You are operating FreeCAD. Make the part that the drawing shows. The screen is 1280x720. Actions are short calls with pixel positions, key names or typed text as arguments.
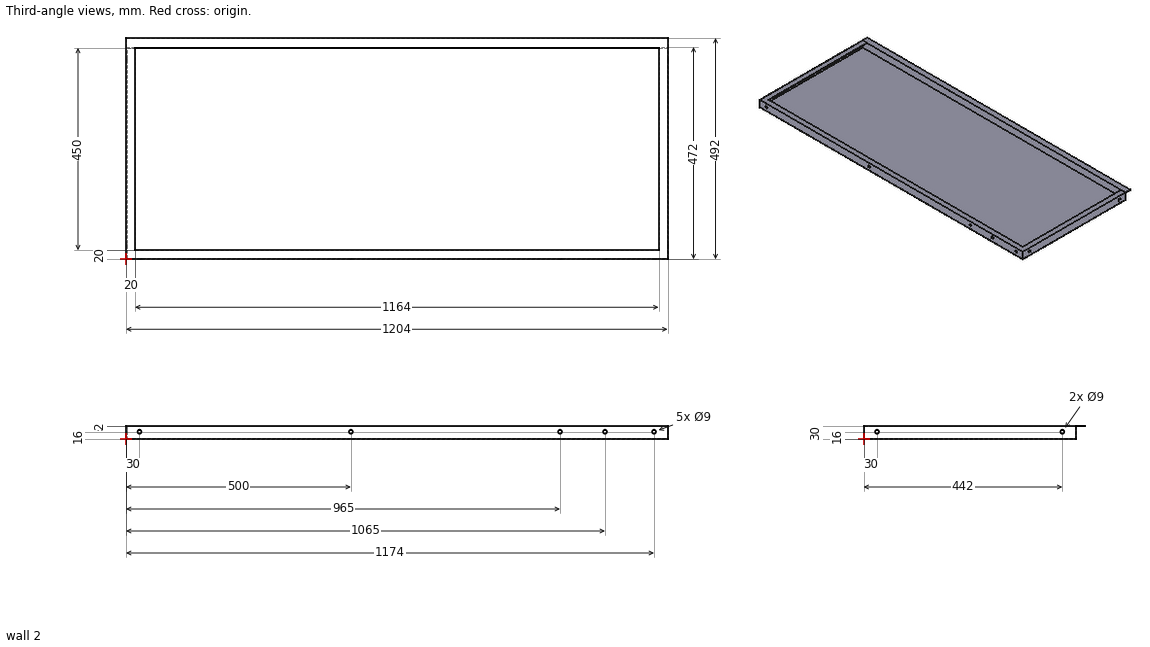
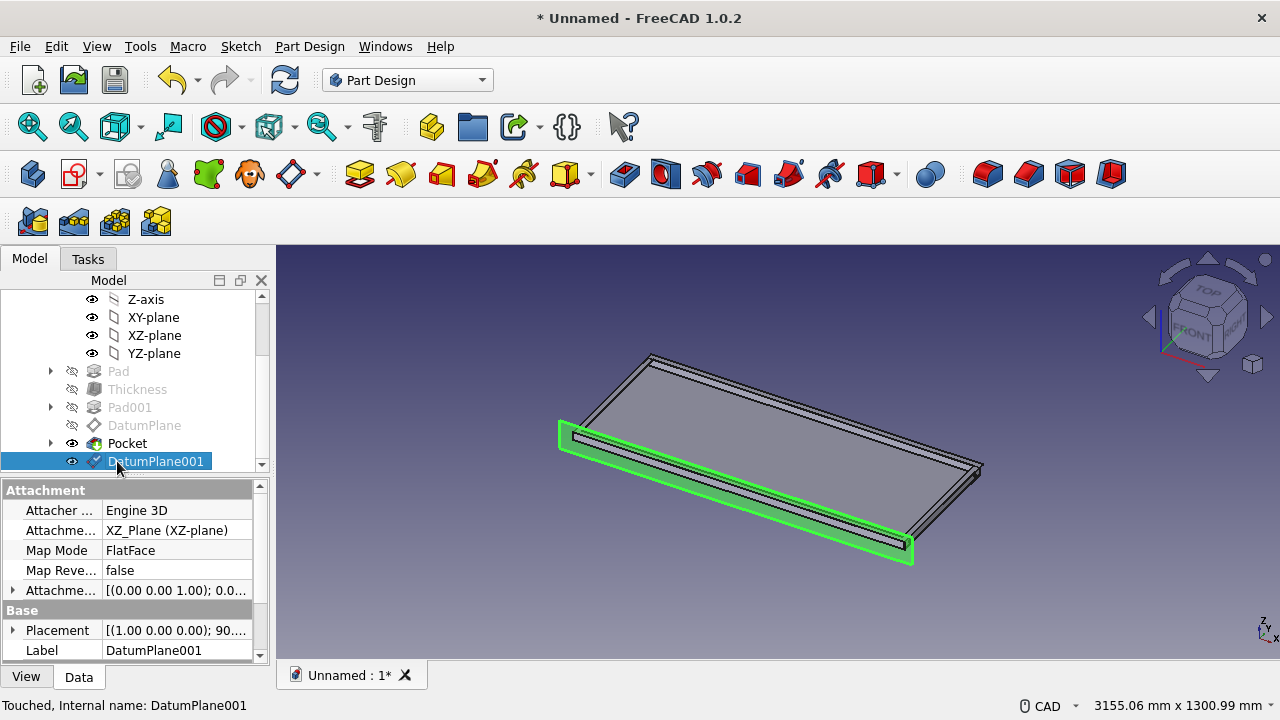
click(74, 174)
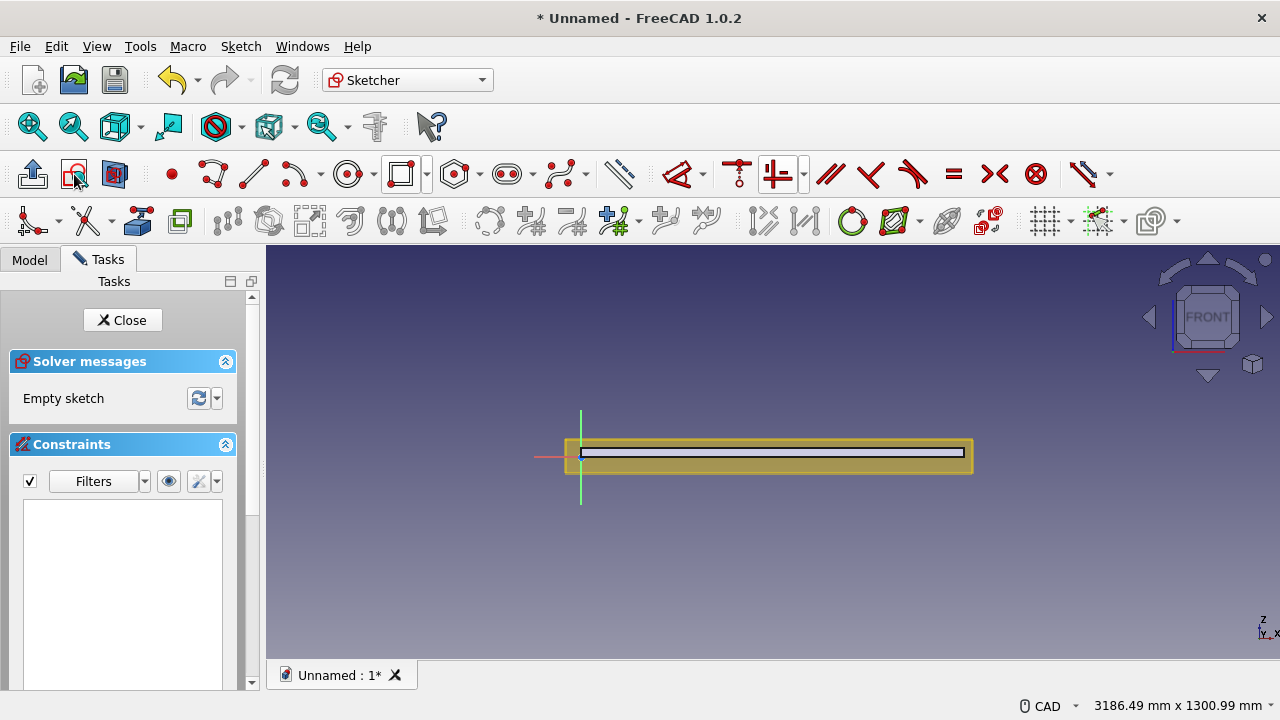
key(q)
key(s)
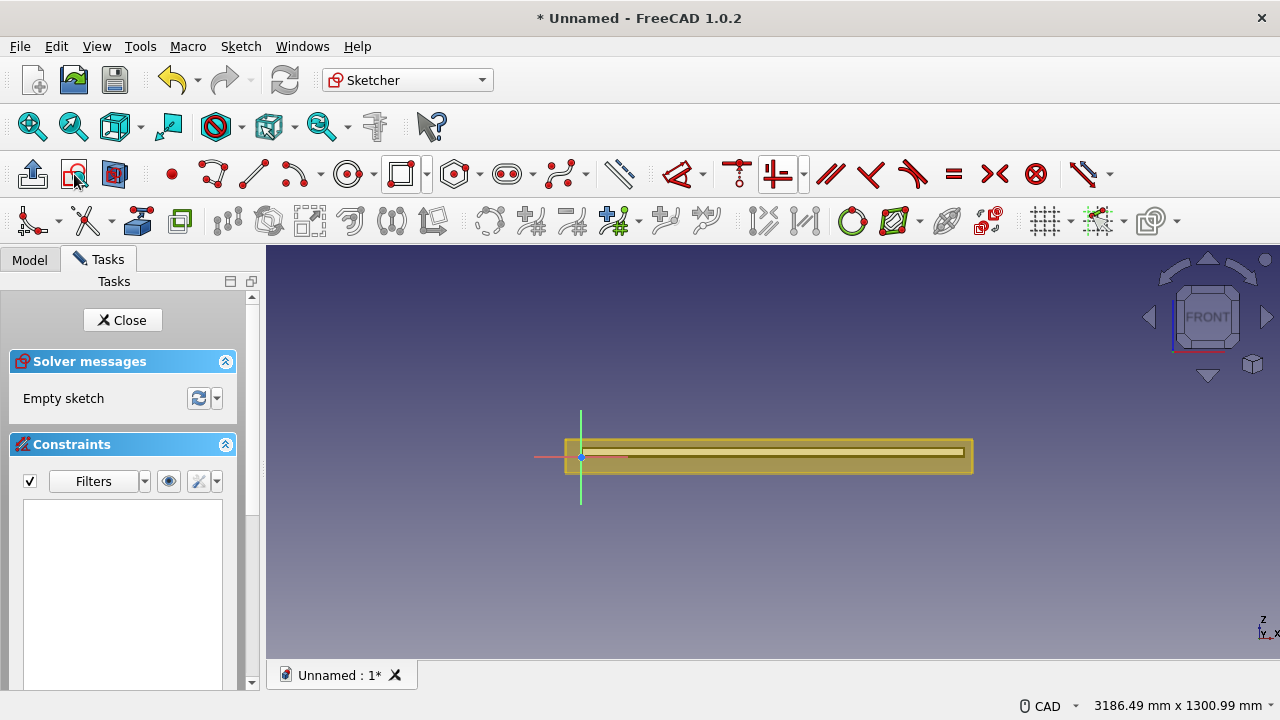
scroll(899, 458, up, 2)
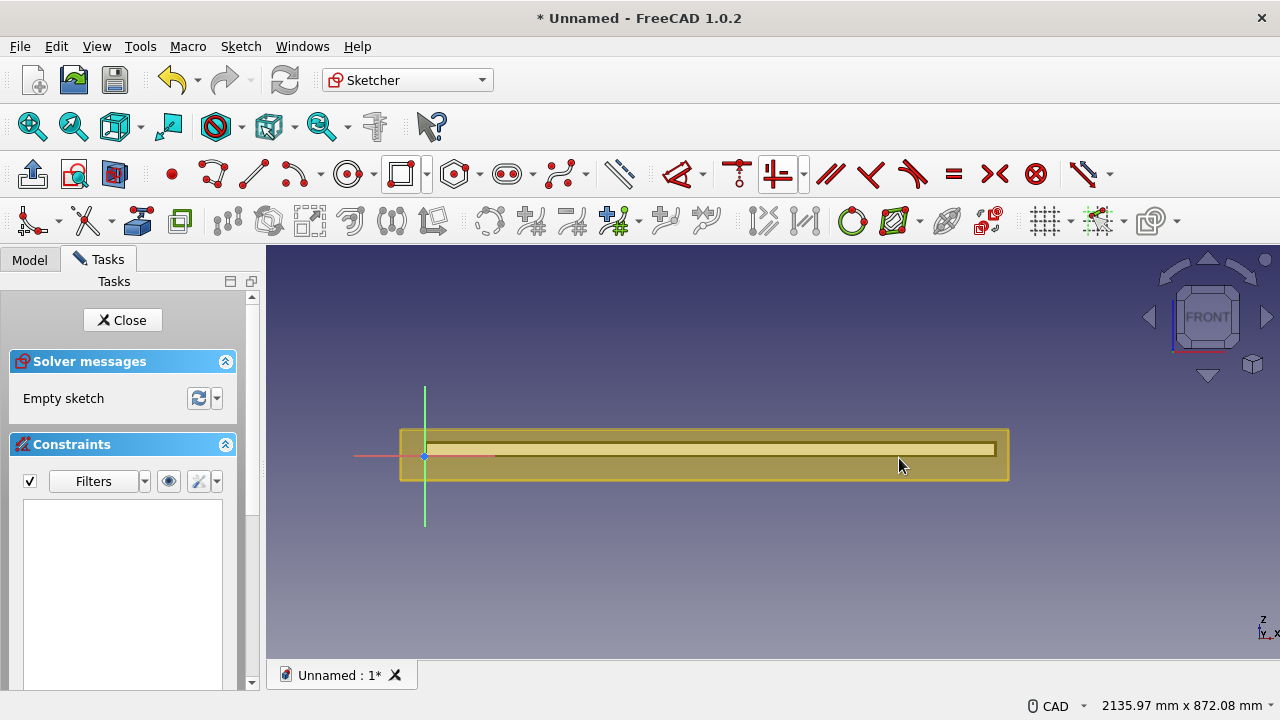
key(g)
key(c)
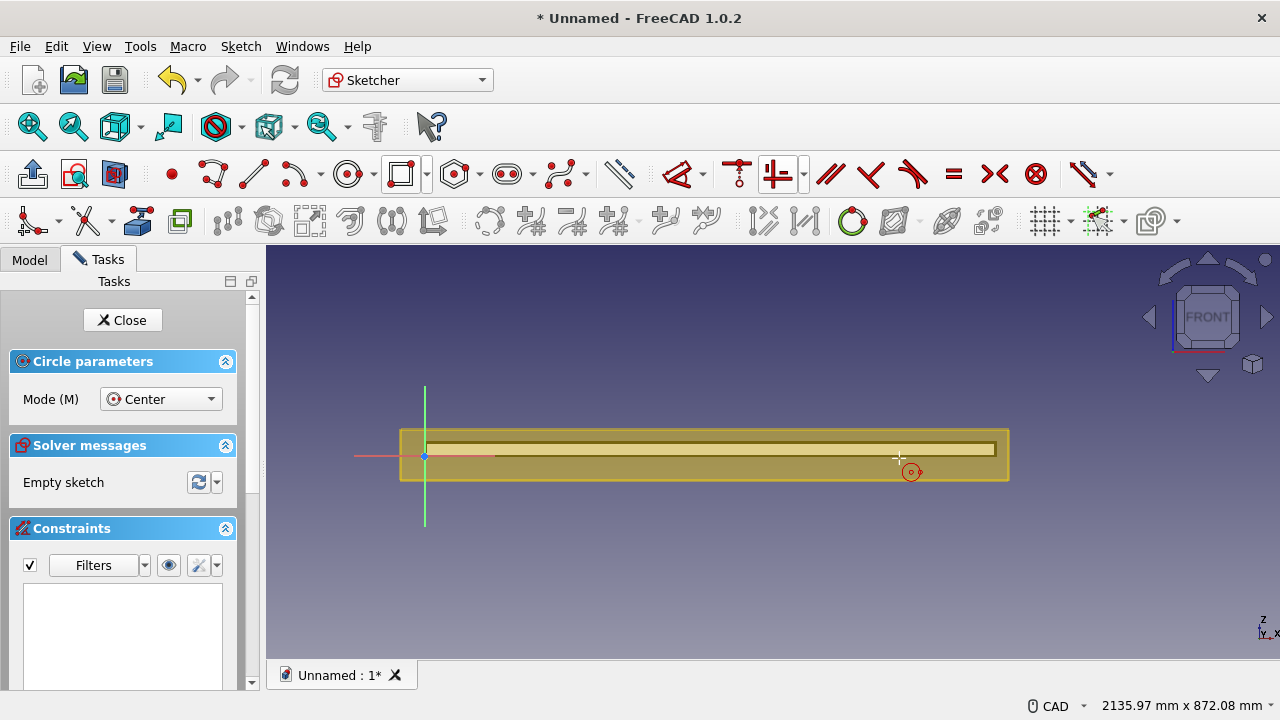
scroll(982, 449, up, 12)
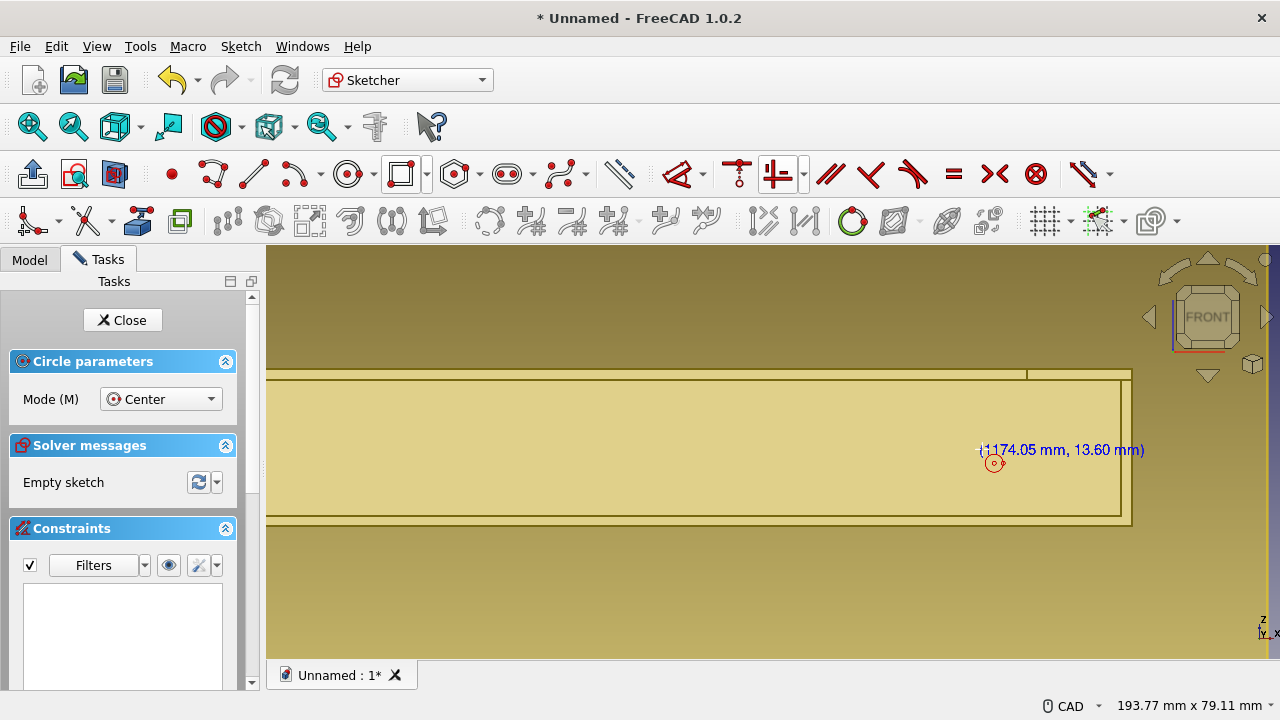
scroll(983, 450, down, 12)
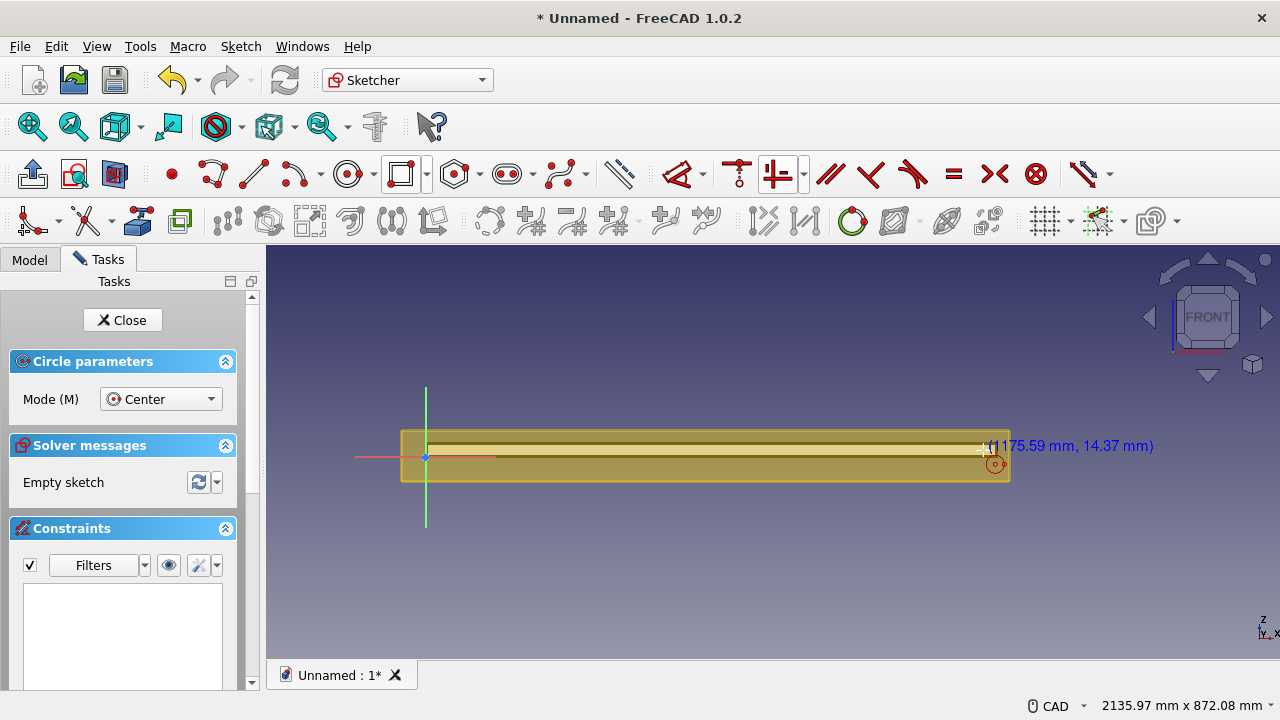
scroll(983, 450, up, 4)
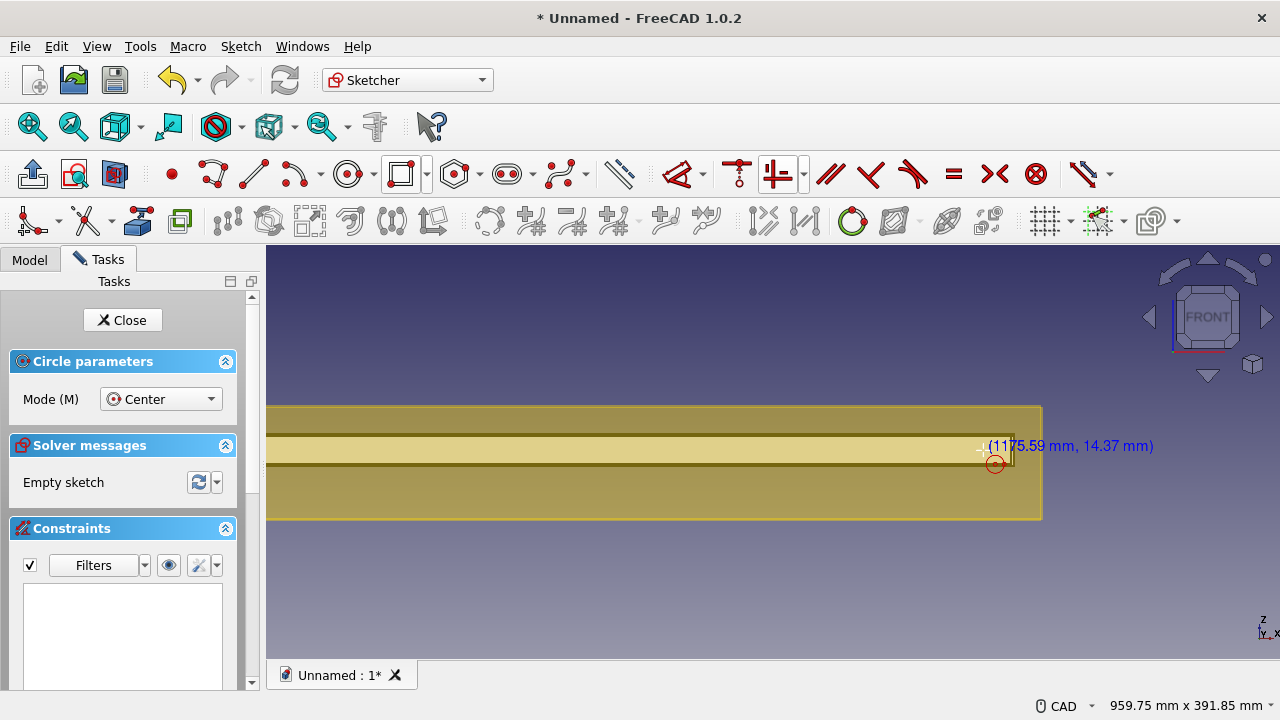
click(982, 449)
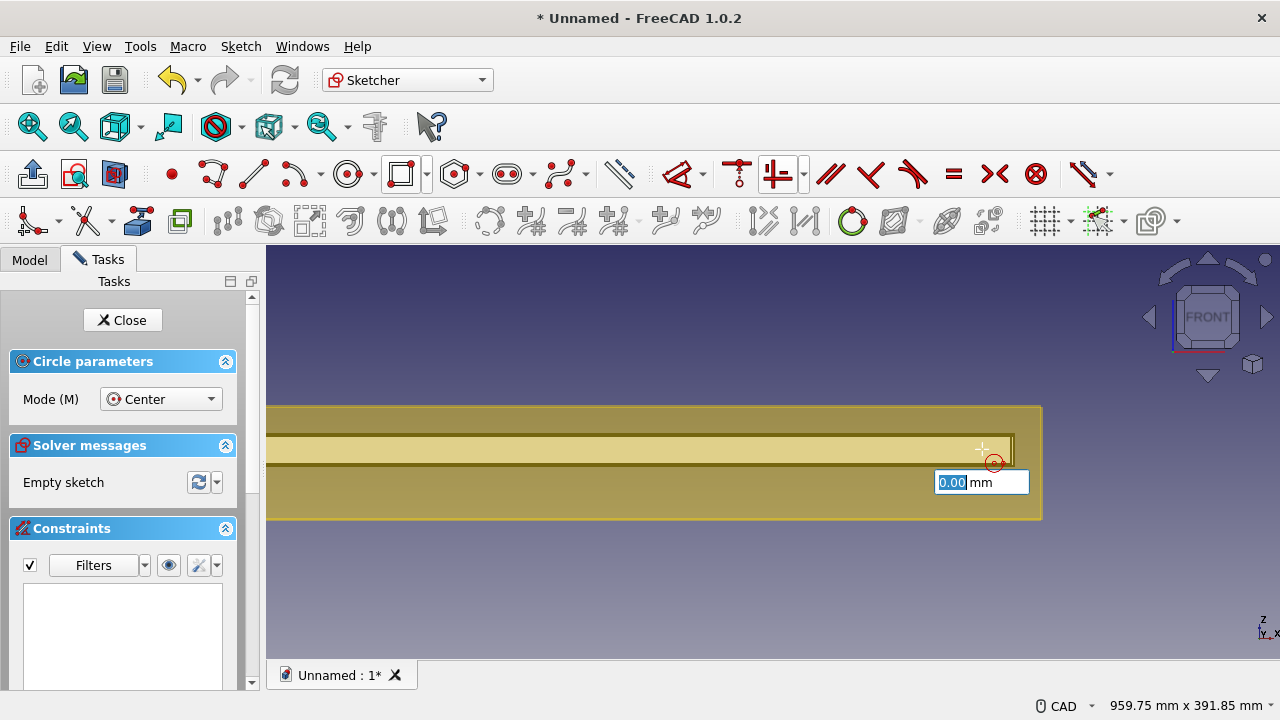
scroll(985, 446, up, 7)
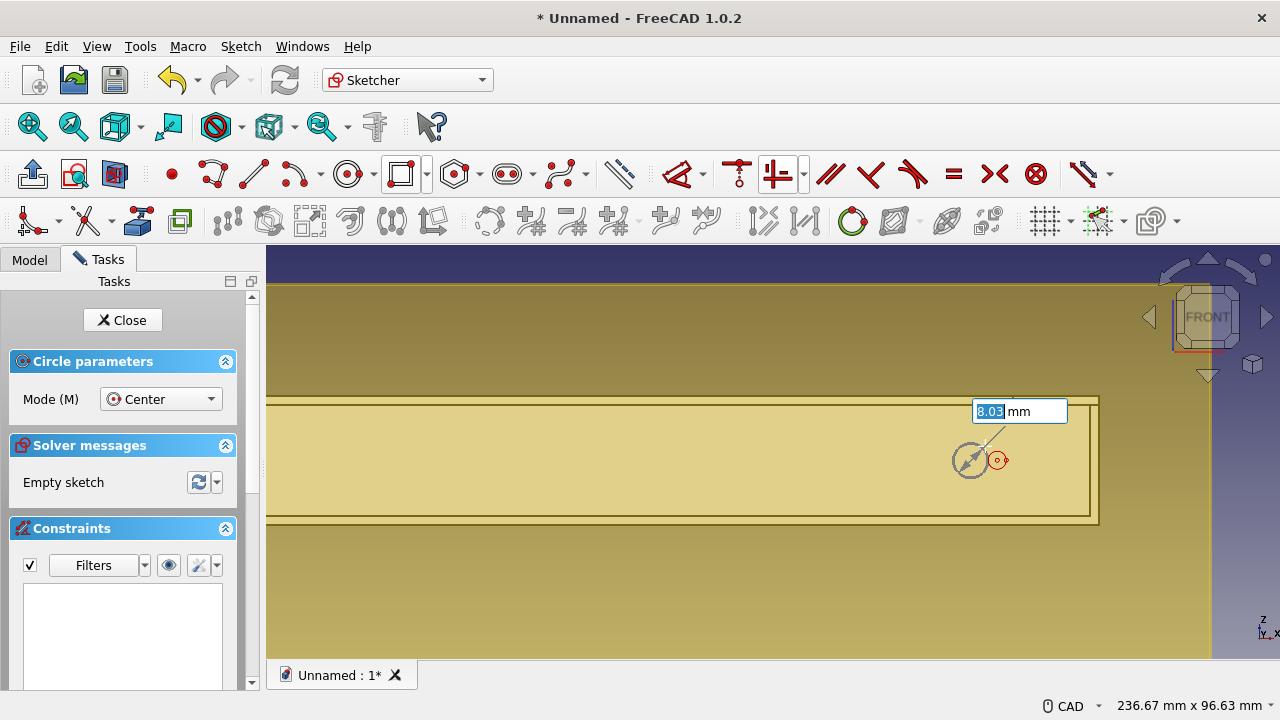
click(984, 443)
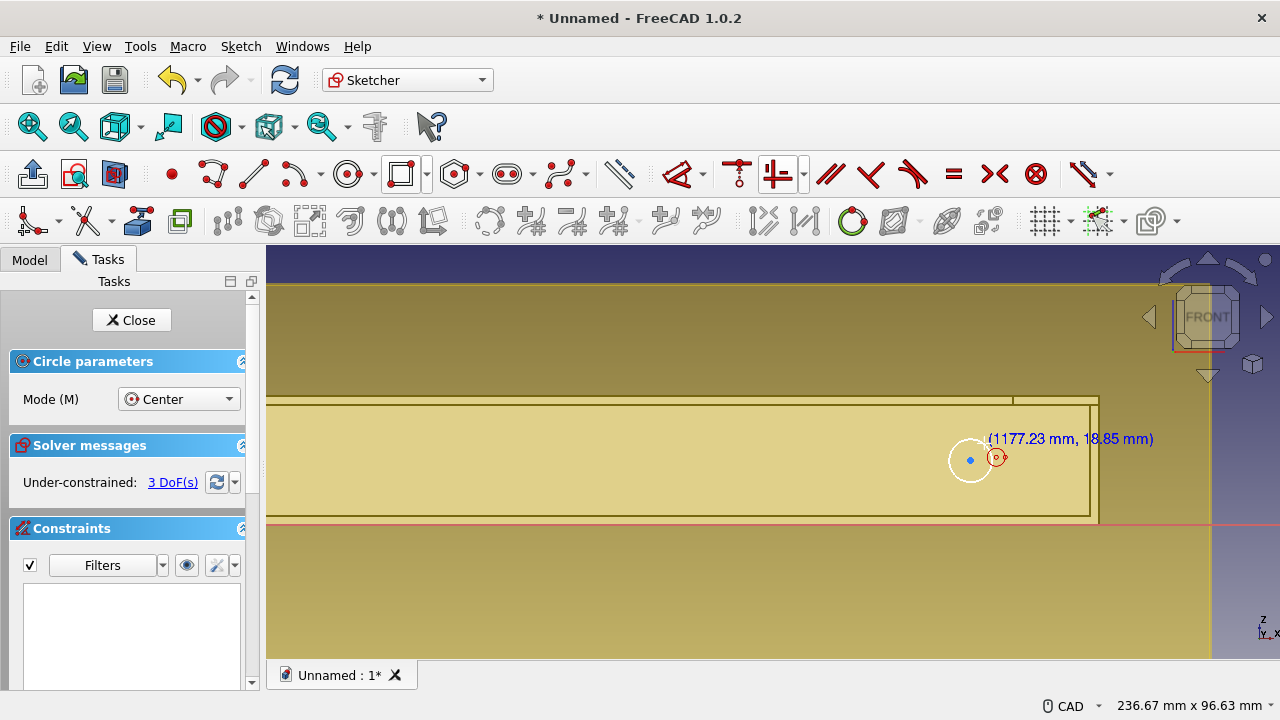
scroll(984, 448, down, 11)